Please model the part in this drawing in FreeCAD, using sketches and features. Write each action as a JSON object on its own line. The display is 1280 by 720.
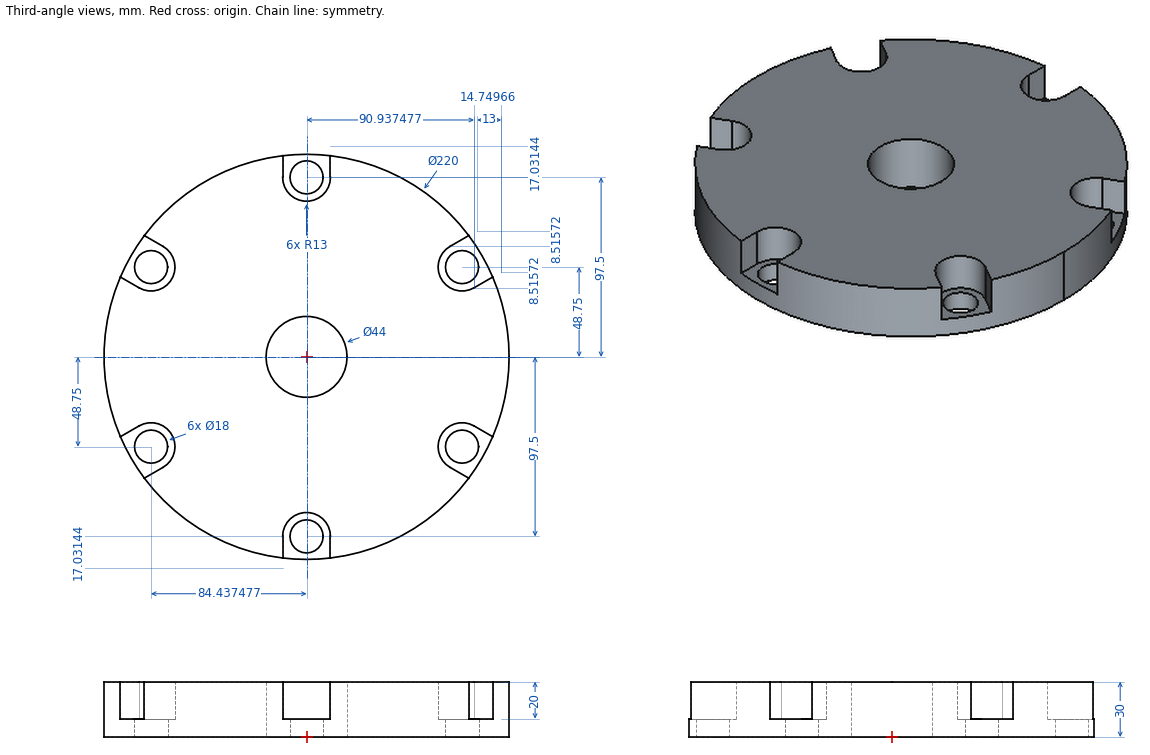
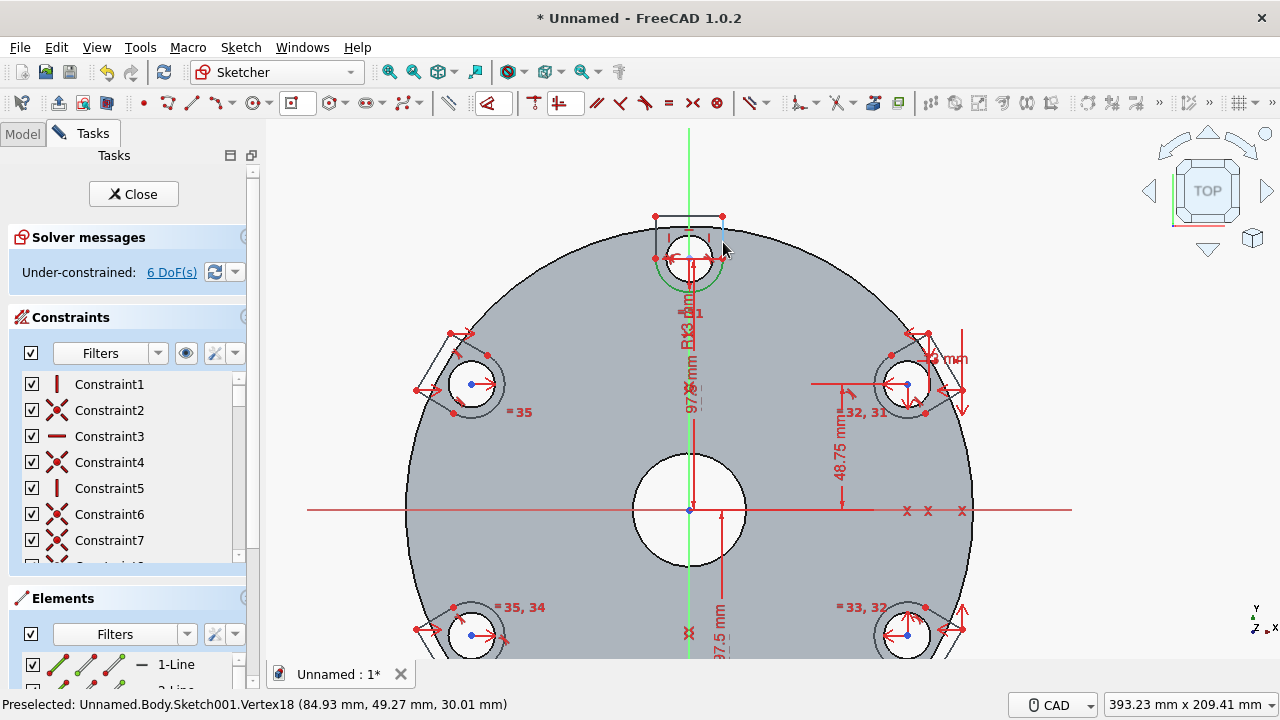
{"action": "left_click", "coordinate": [723, 242]}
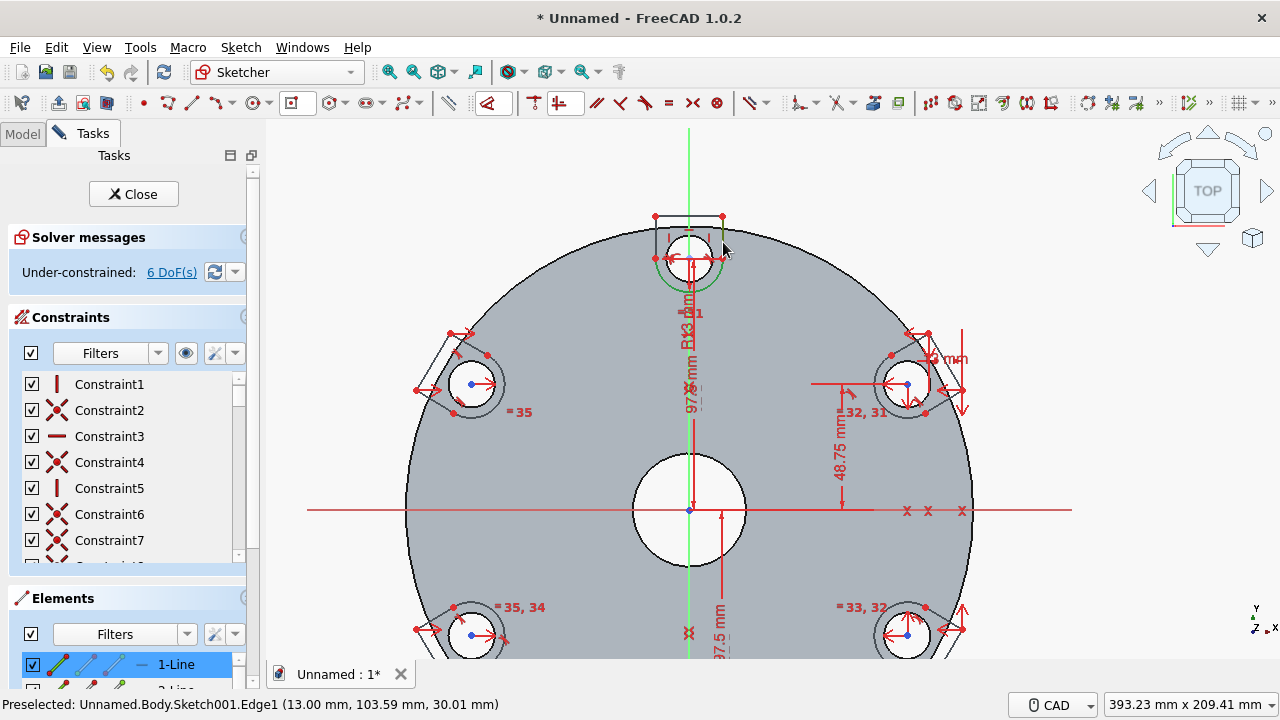
{"action": "key", "text": "i"}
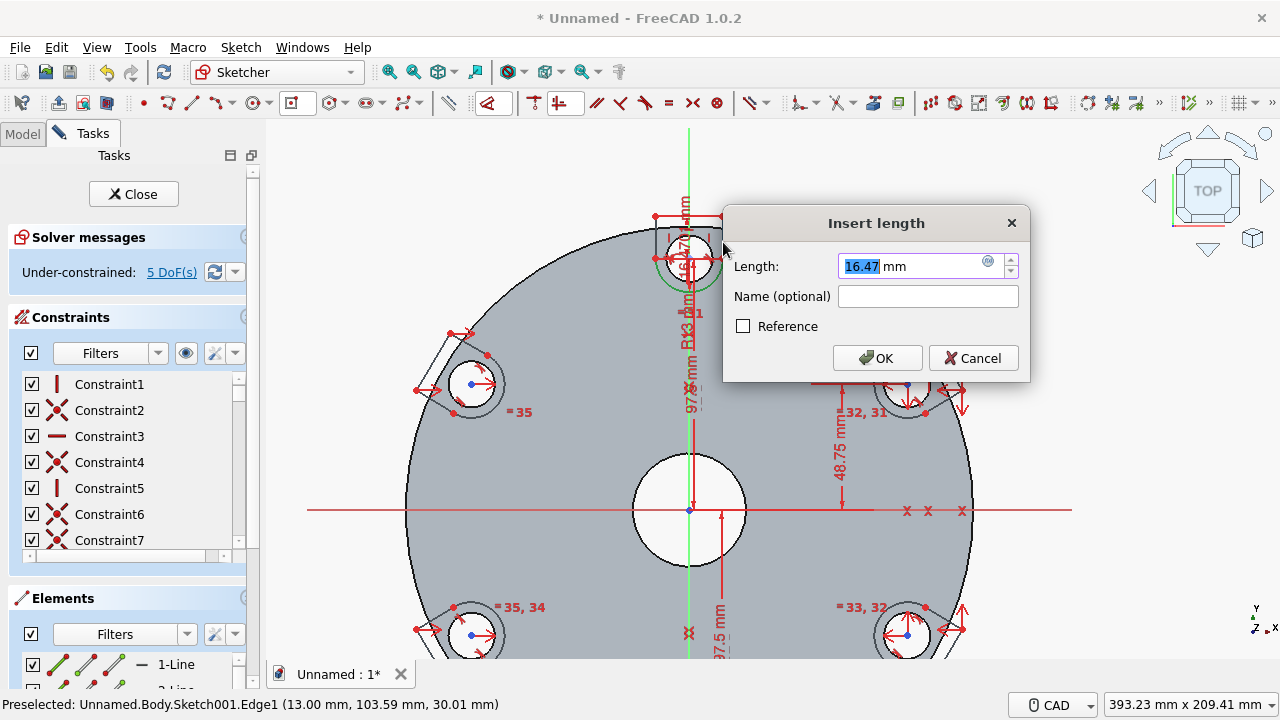
{"action": "type", "text": "17.03144"}
{"action": "key", "text": "Return"}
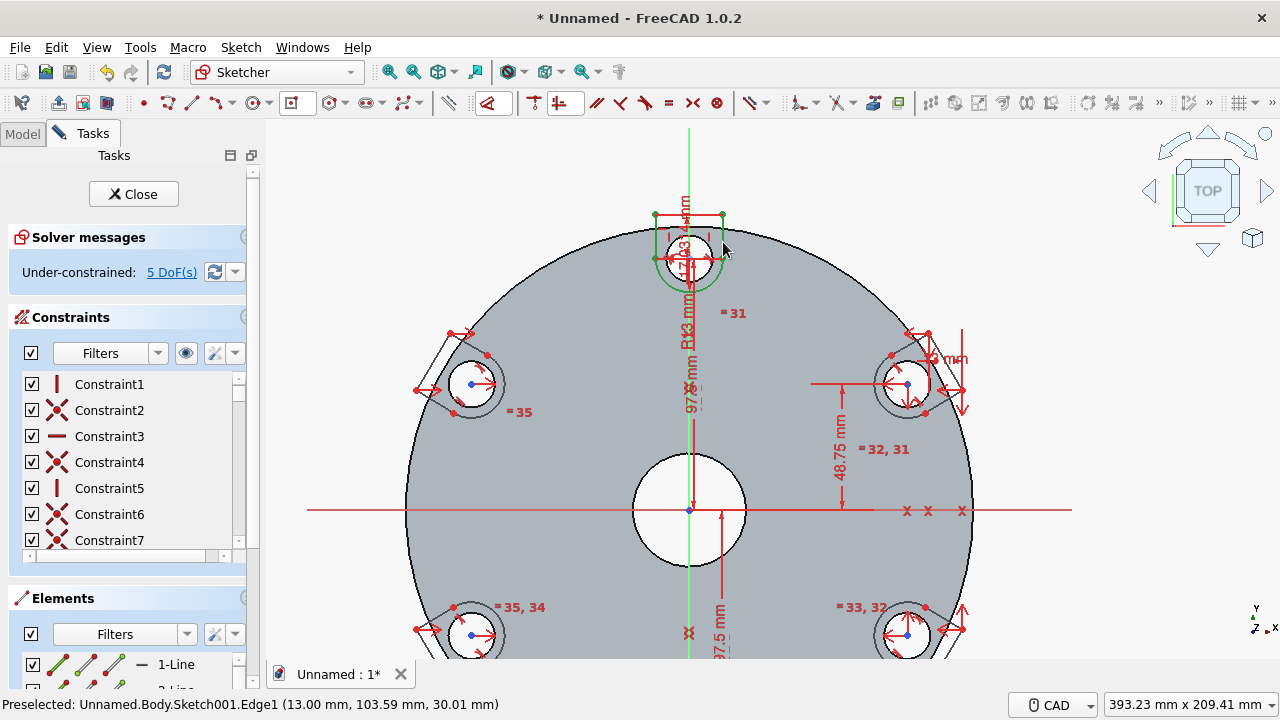
{"action": "scroll", "coordinate": [723, 242], "scroll_direction": "down", "scroll_amount": 3}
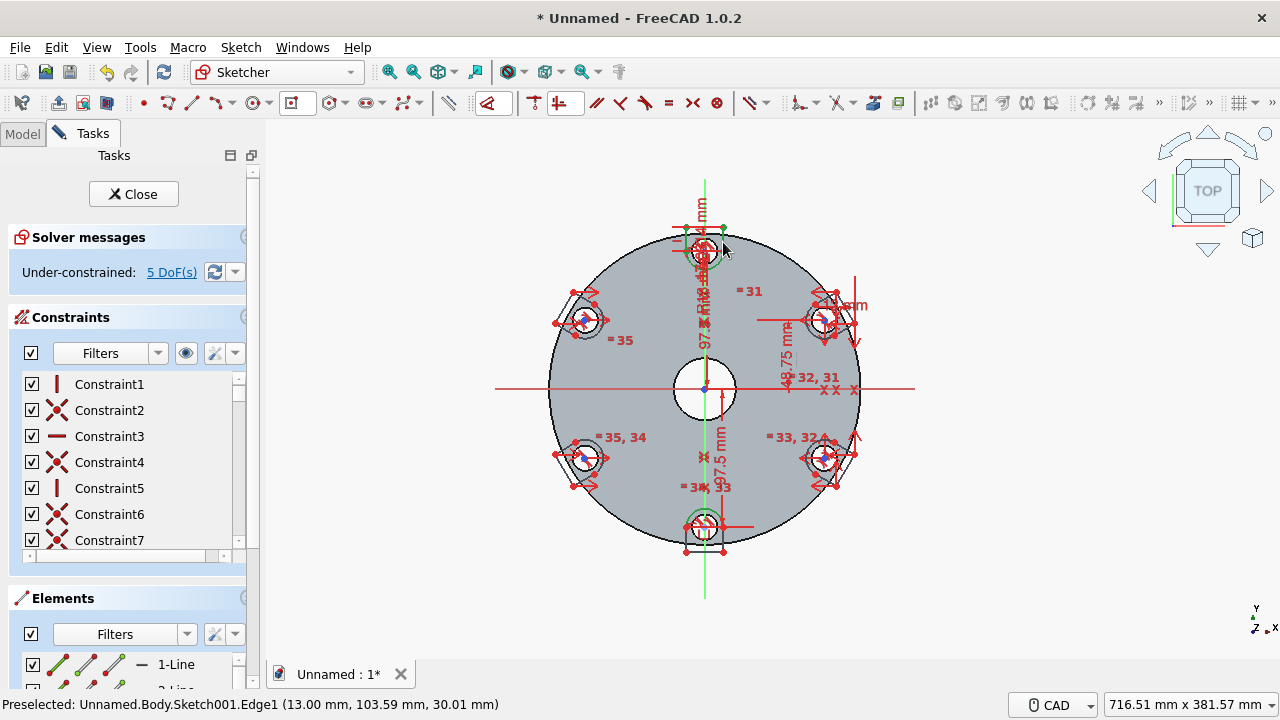
{"action": "scroll", "coordinate": [686, 535], "scroll_direction": "up", "scroll_amount": 4}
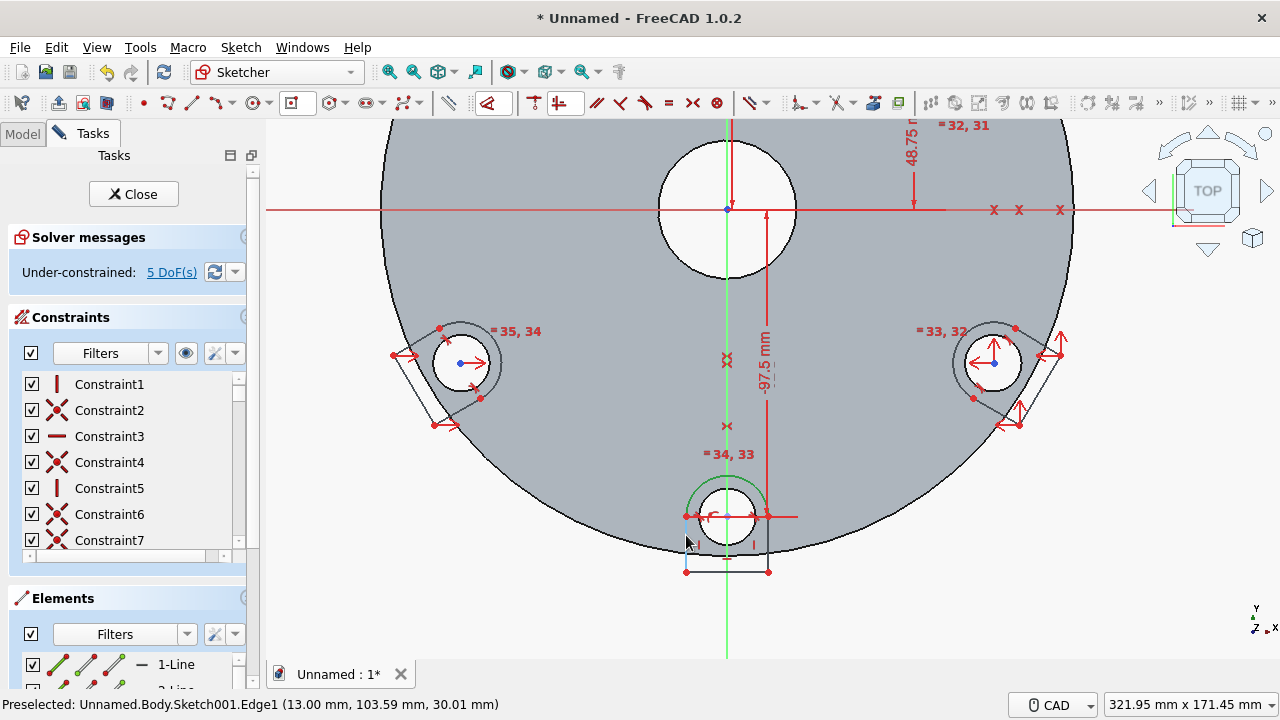
{"action": "left_click", "coordinate": [686, 533]}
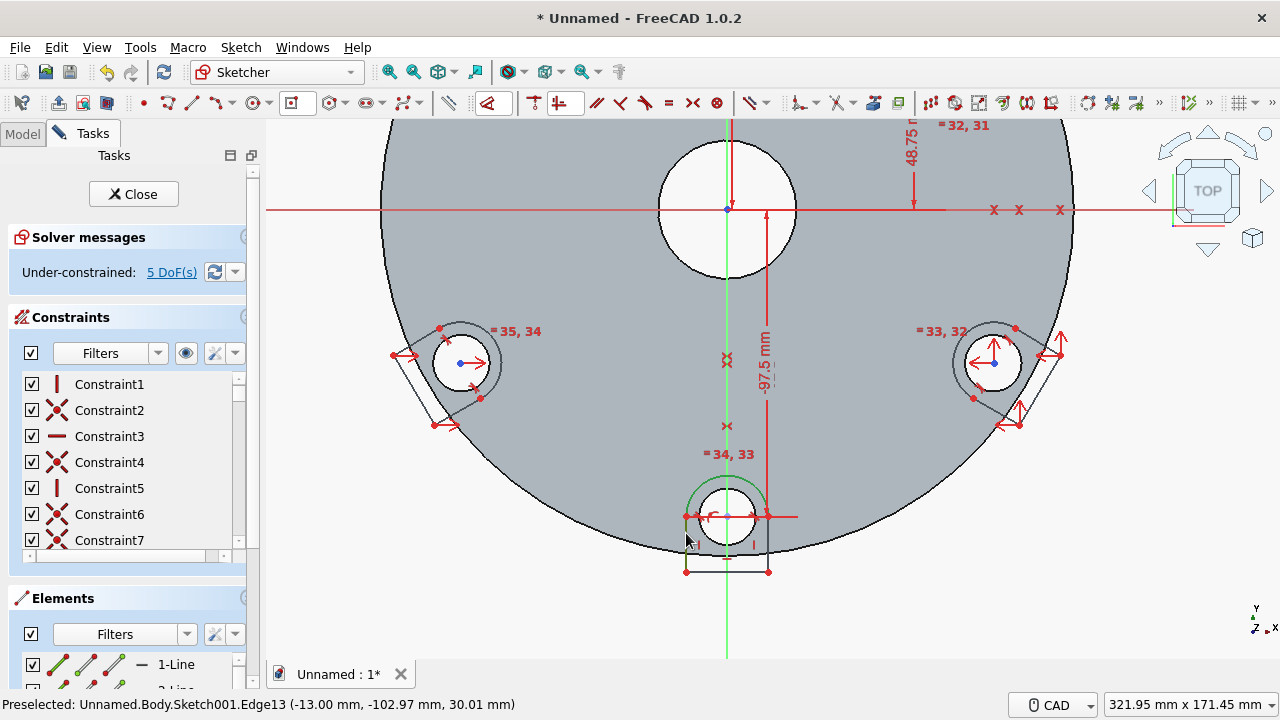
{"action": "key", "text": "i"}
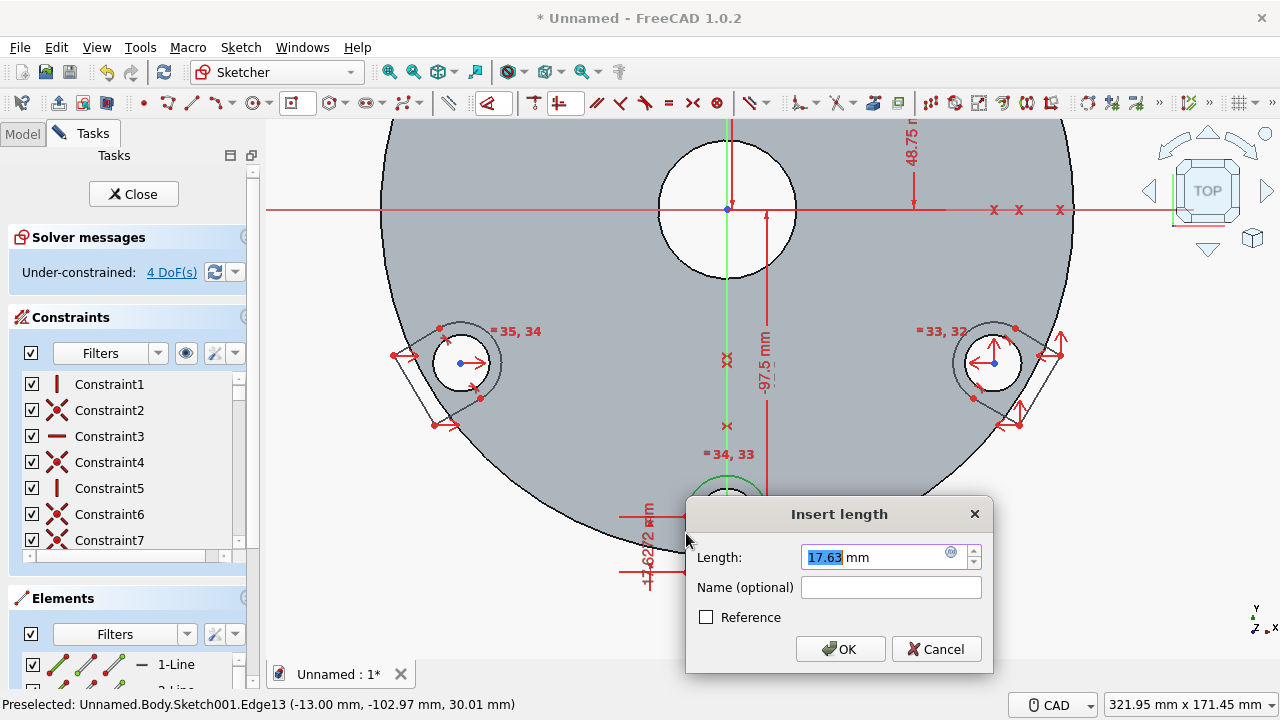
{"action": "type", "text": "17.03144"}
{"action": "key", "text": "Return"}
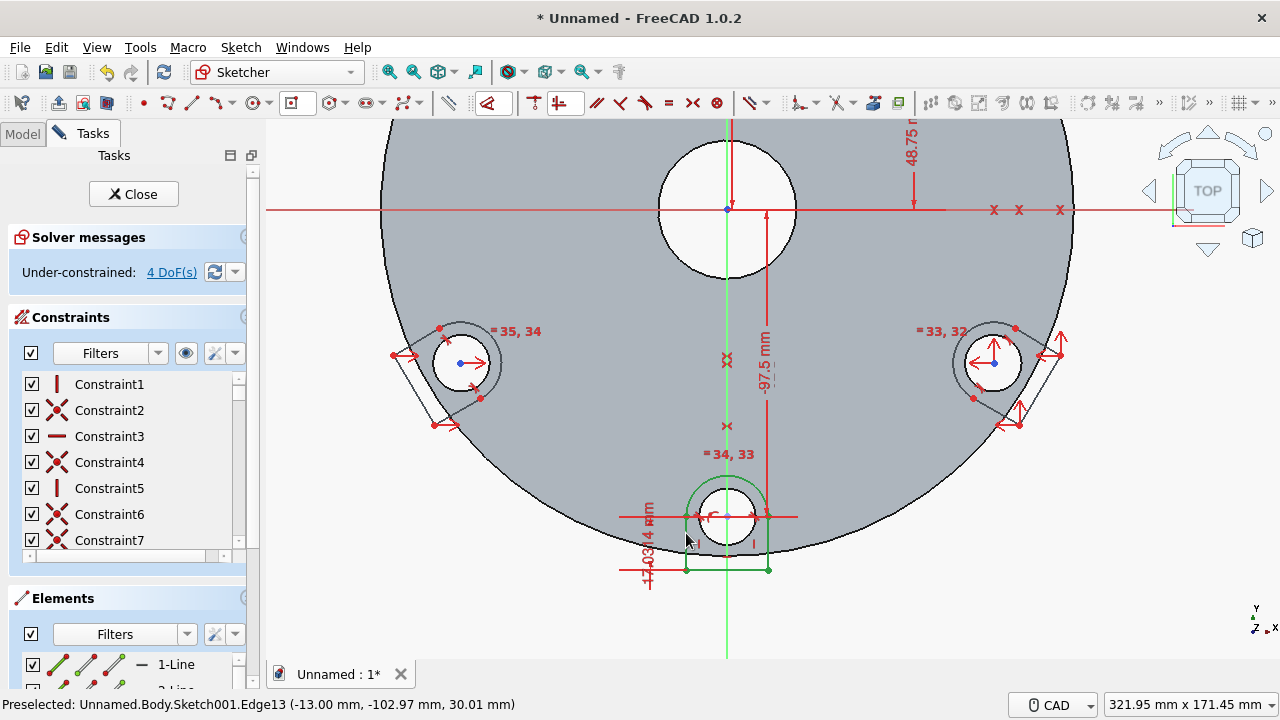
{"action": "scroll", "coordinate": [686, 535], "scroll_direction": "down", "scroll_amount": 4}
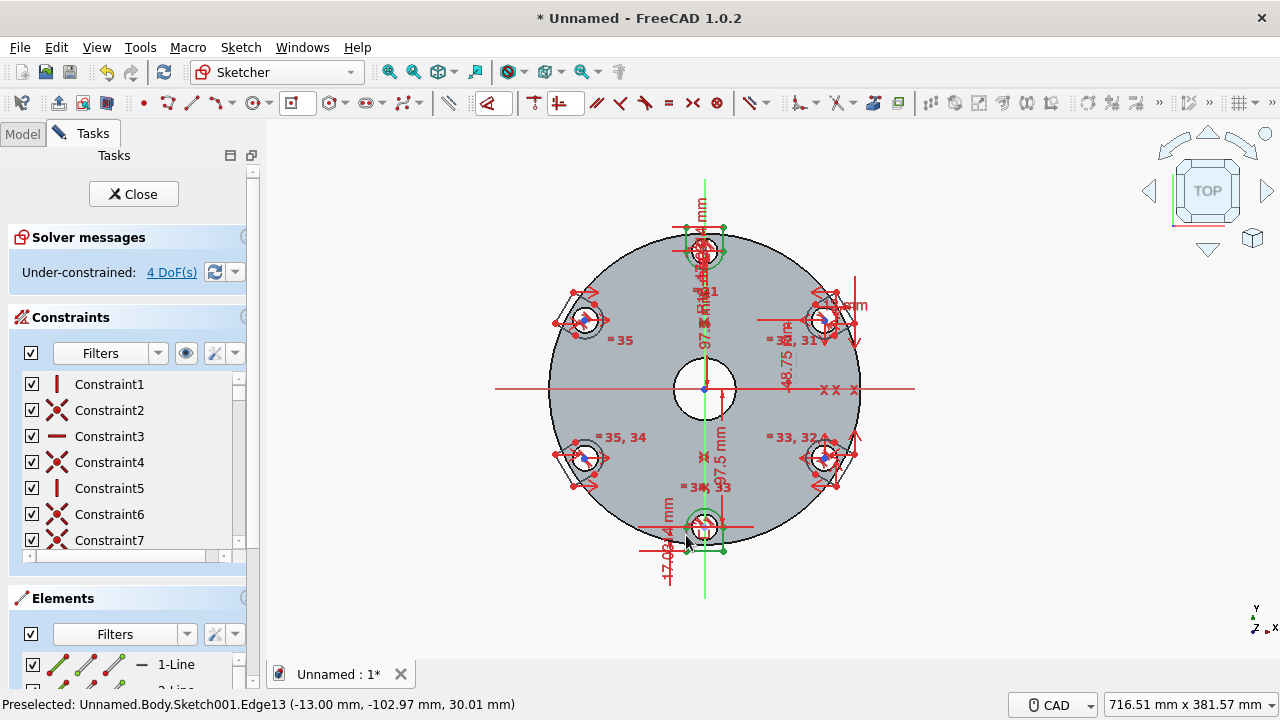
{"action": "scroll", "coordinate": [840, 332], "scroll_direction": "up", "scroll_amount": 6}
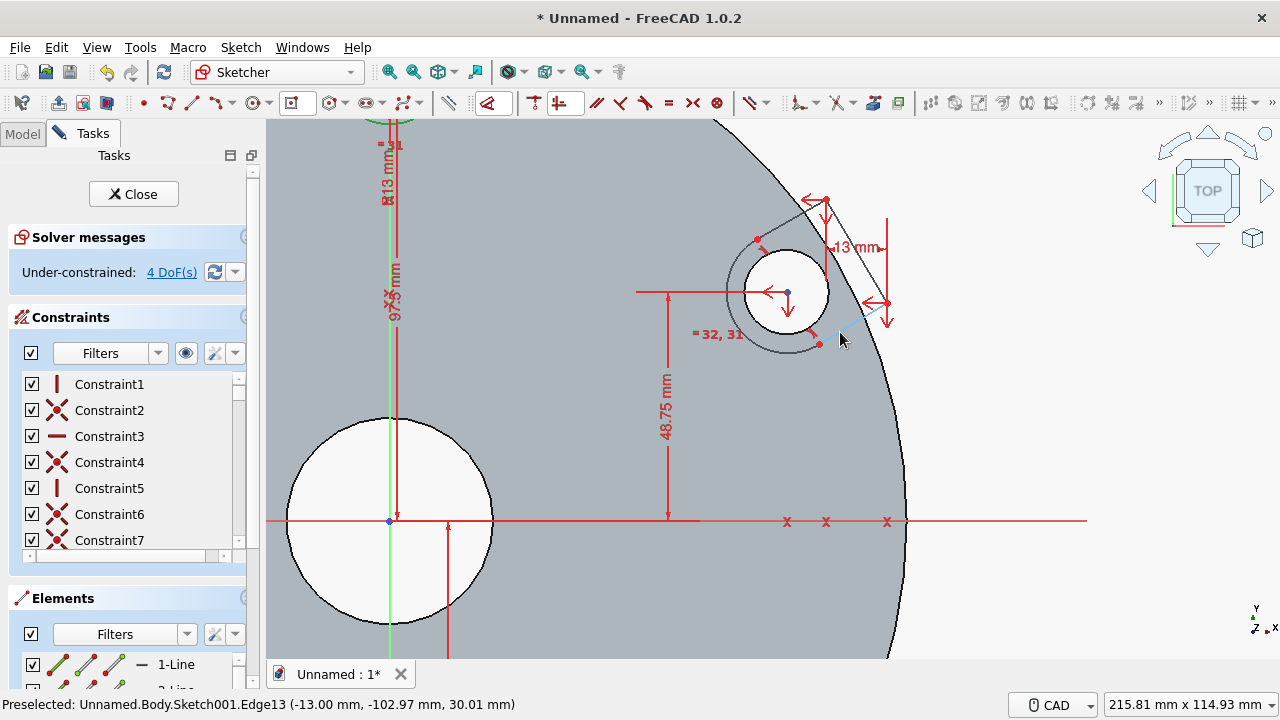
{"action": "left_click", "coordinate": [840, 332]}